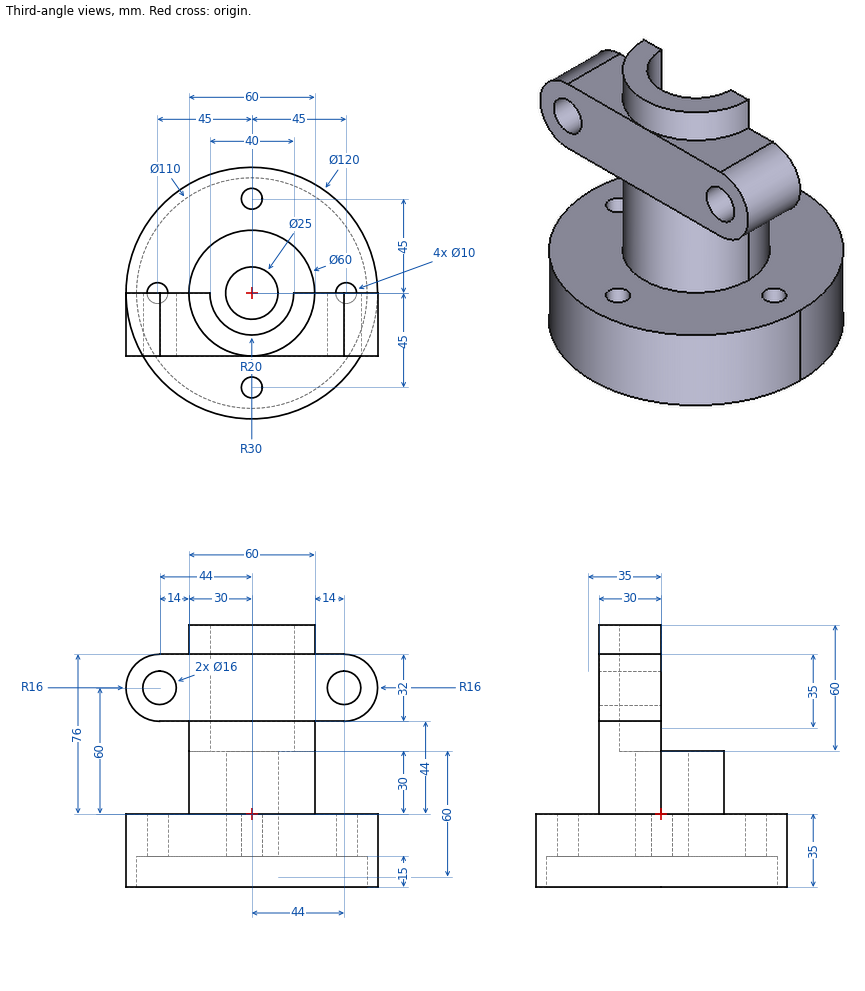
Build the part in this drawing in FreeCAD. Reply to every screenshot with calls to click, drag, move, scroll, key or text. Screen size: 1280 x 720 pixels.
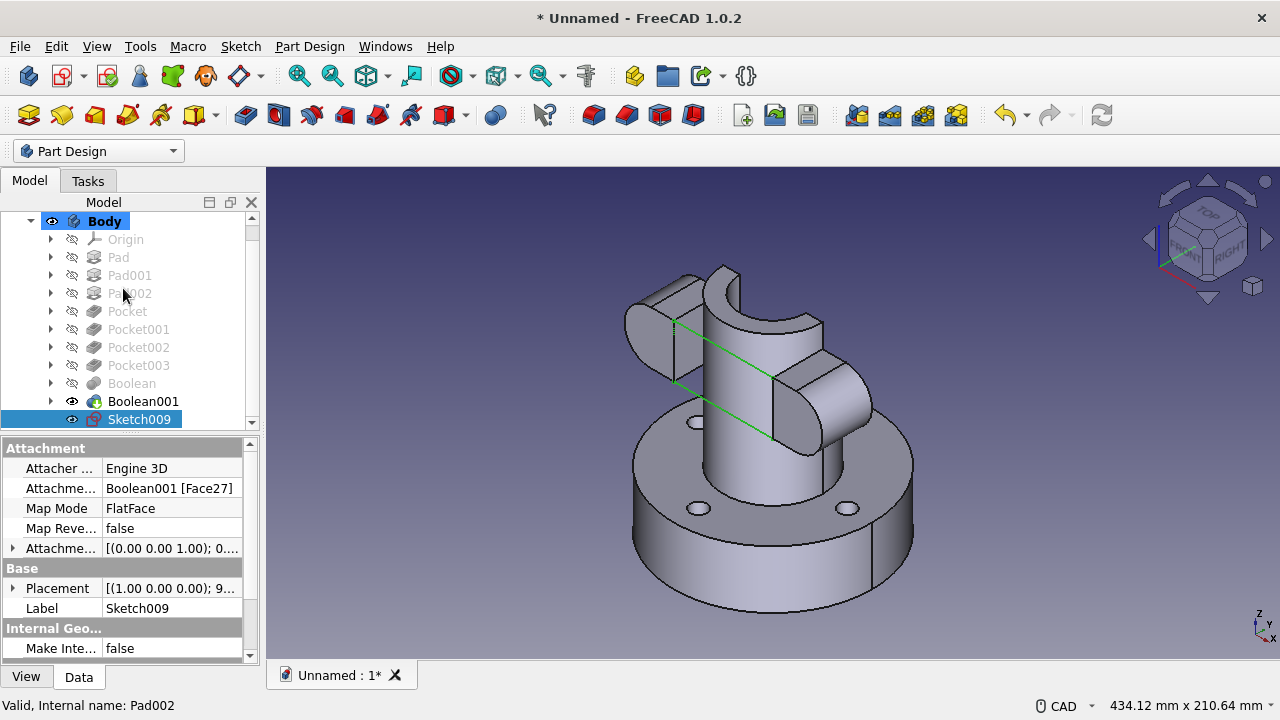
click(29, 116)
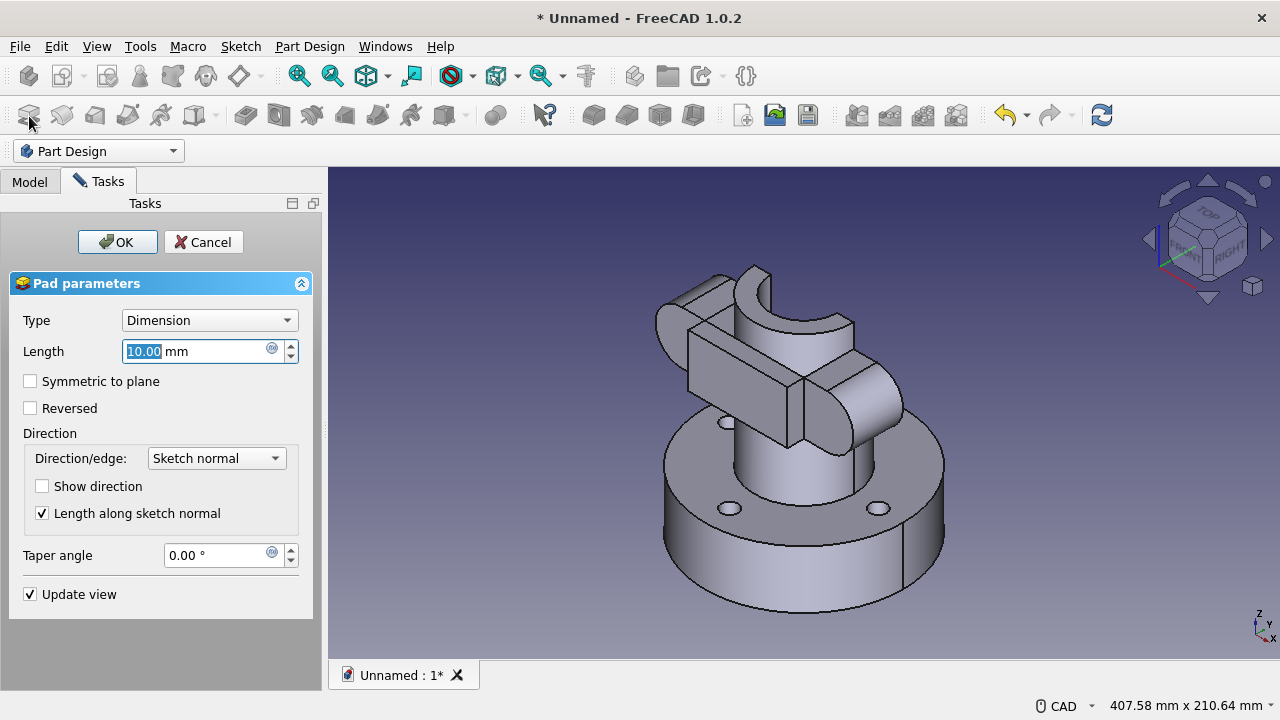
text(30)
key(Tab)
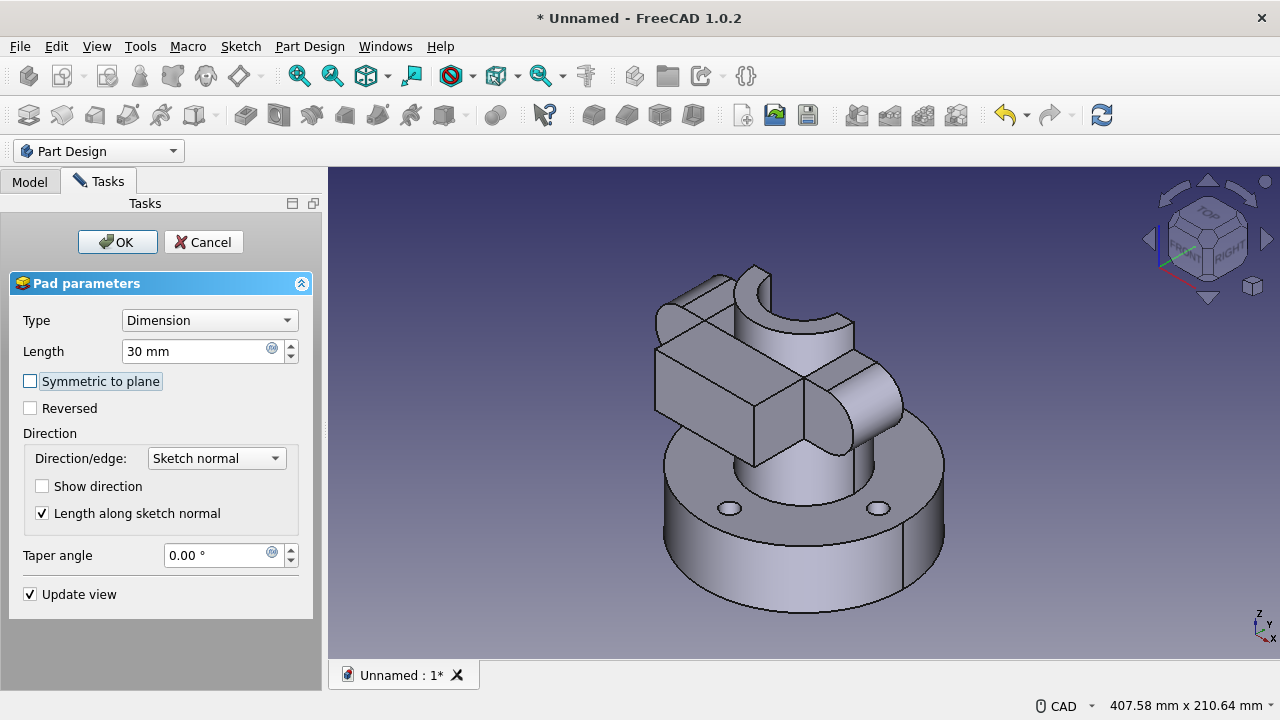
click(31, 408)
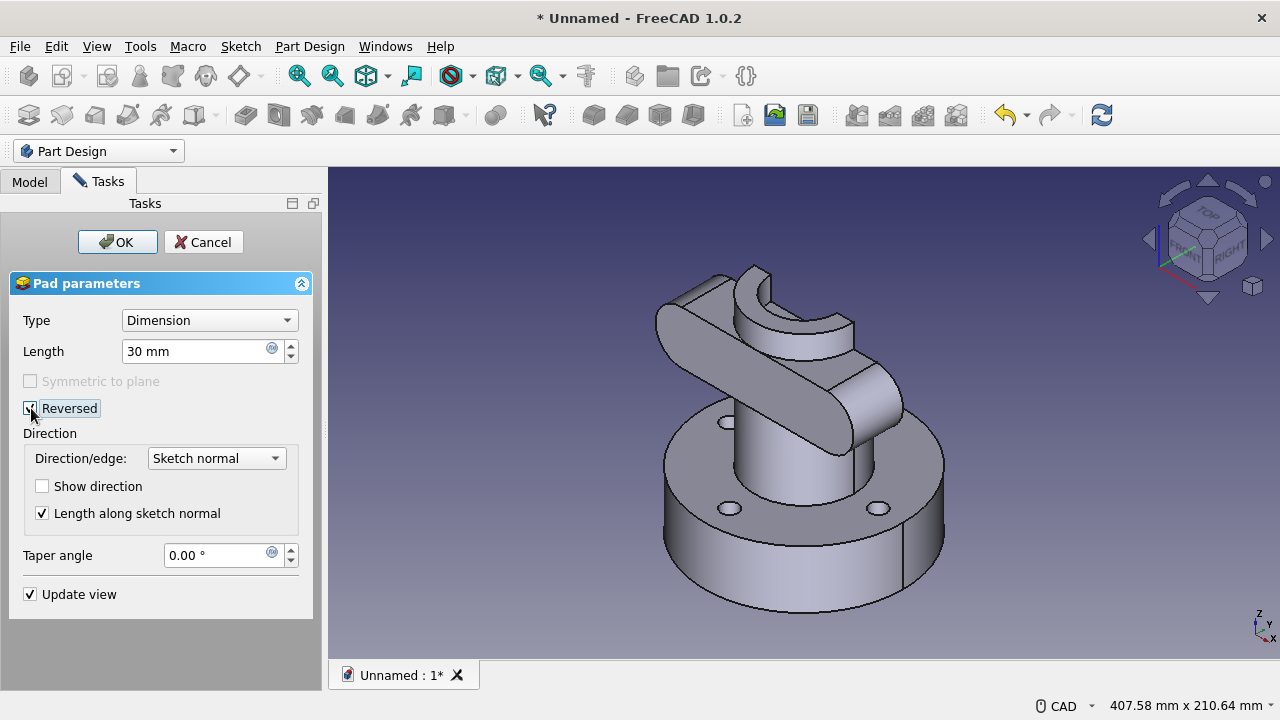
click(118, 242)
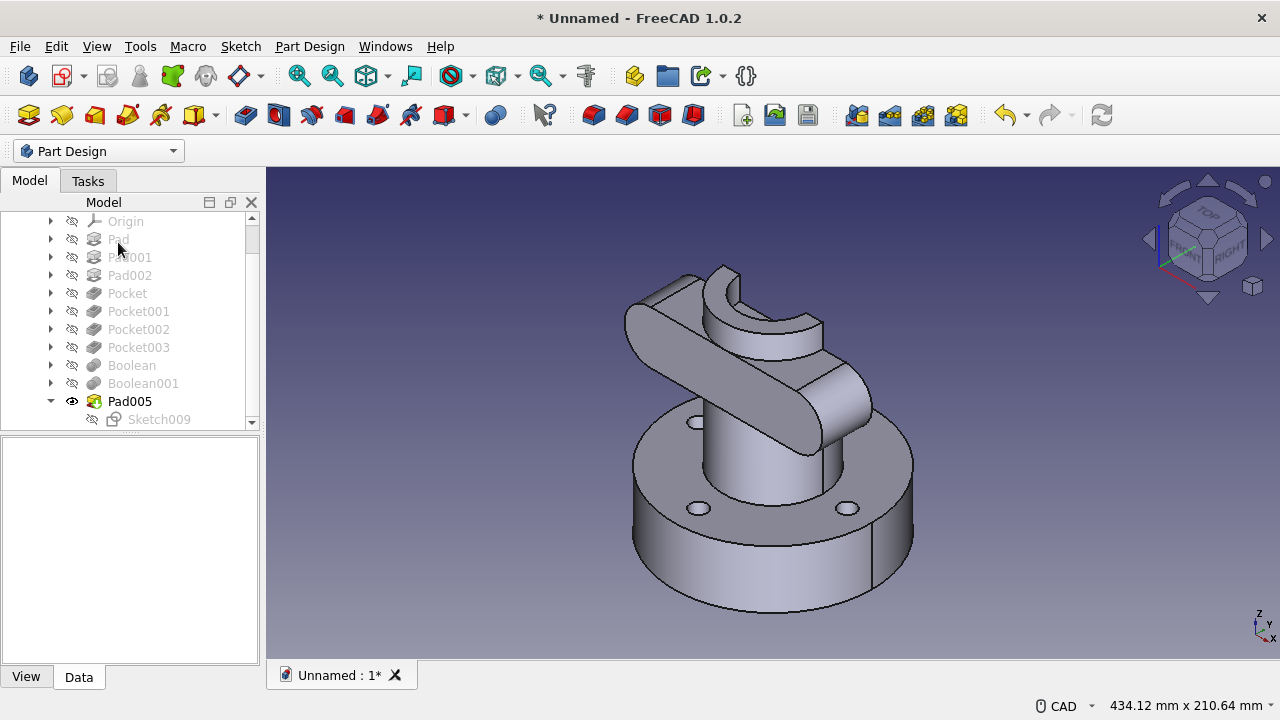
key(2)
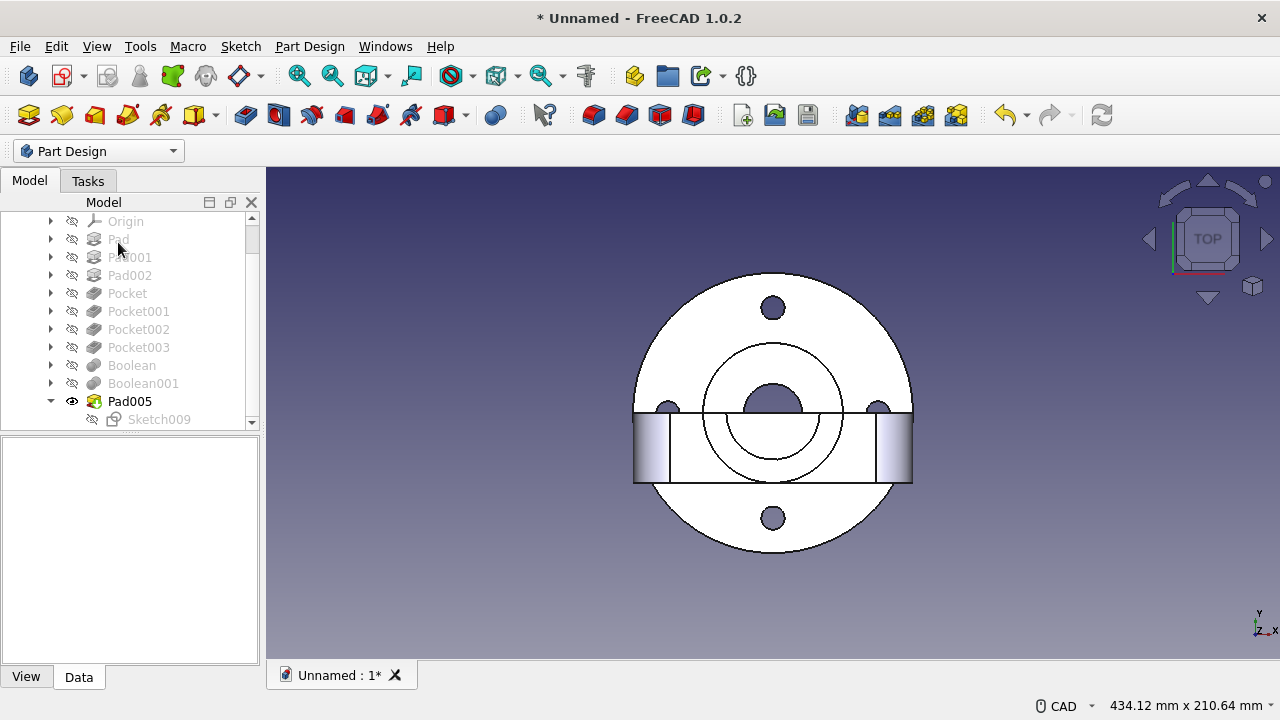
click(773, 435)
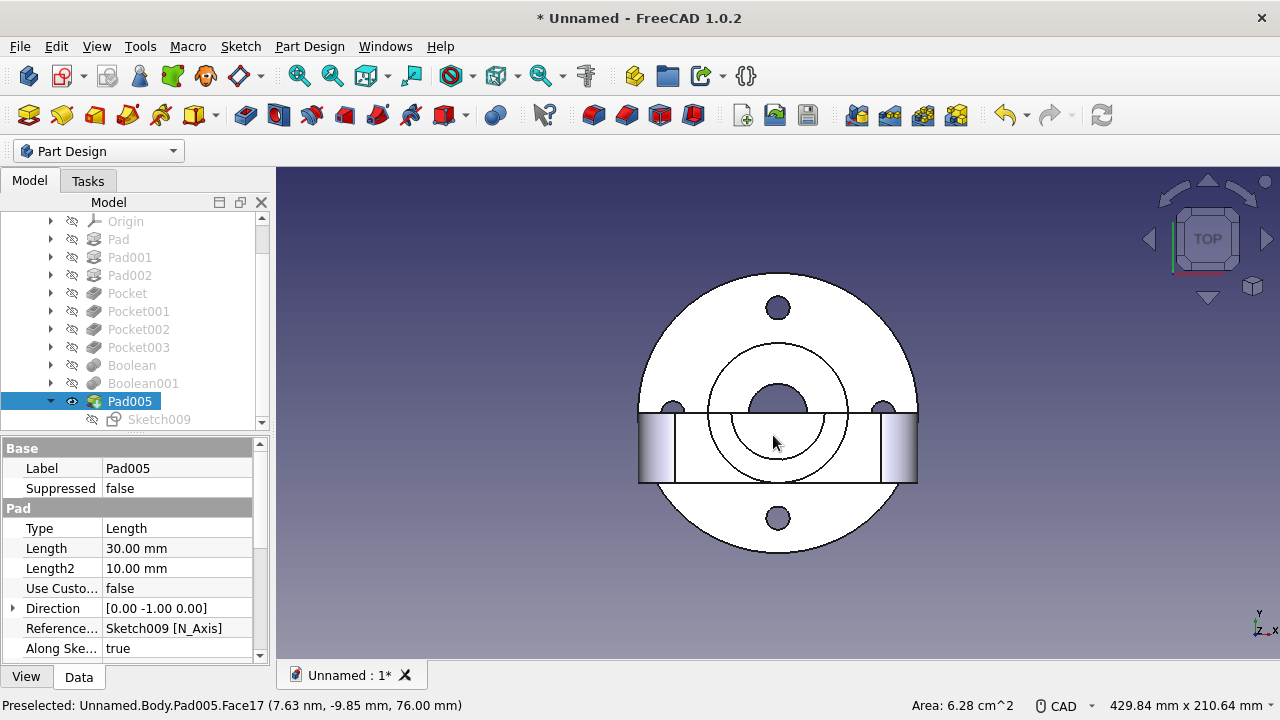
click(62, 76)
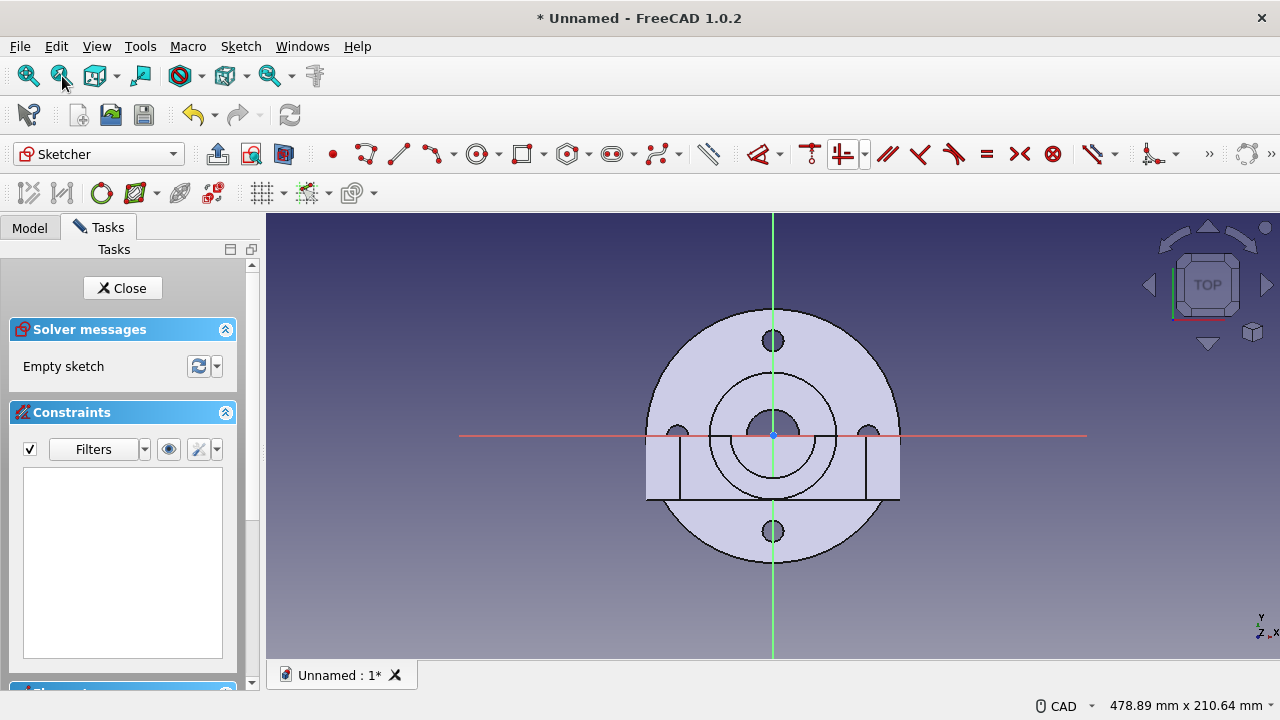
scroll(787, 461, up, 9)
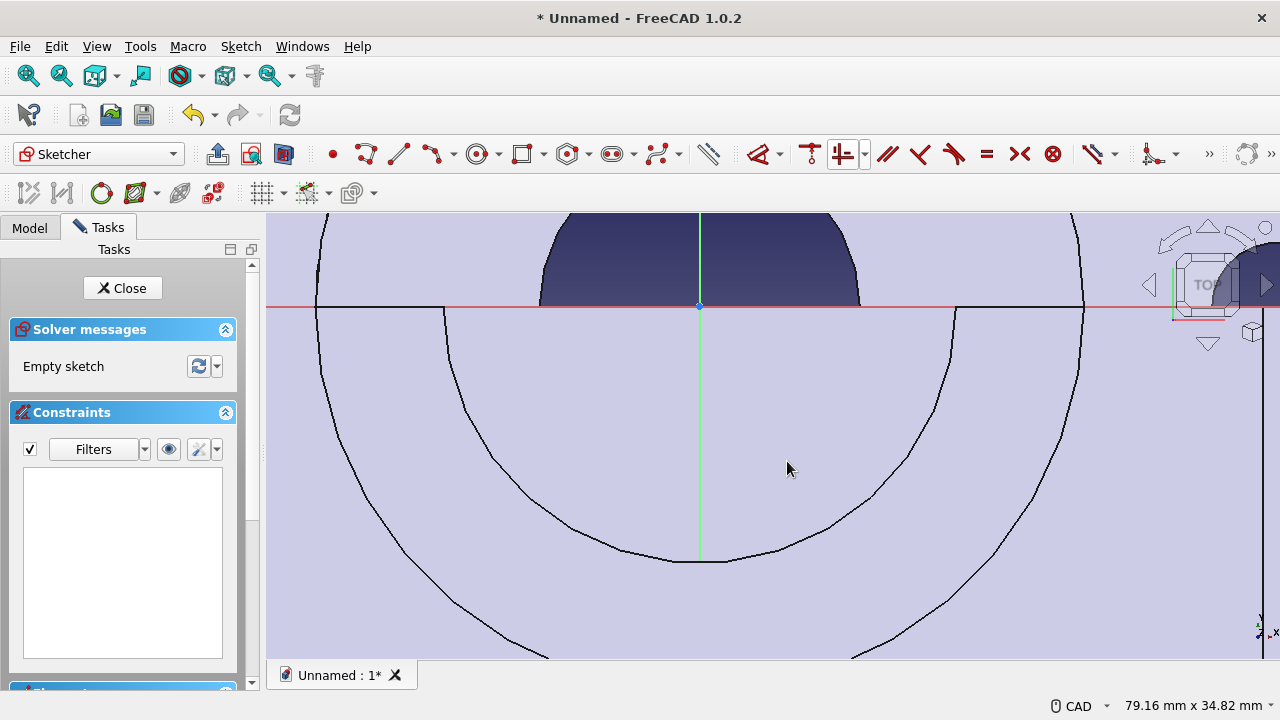
click(399, 154)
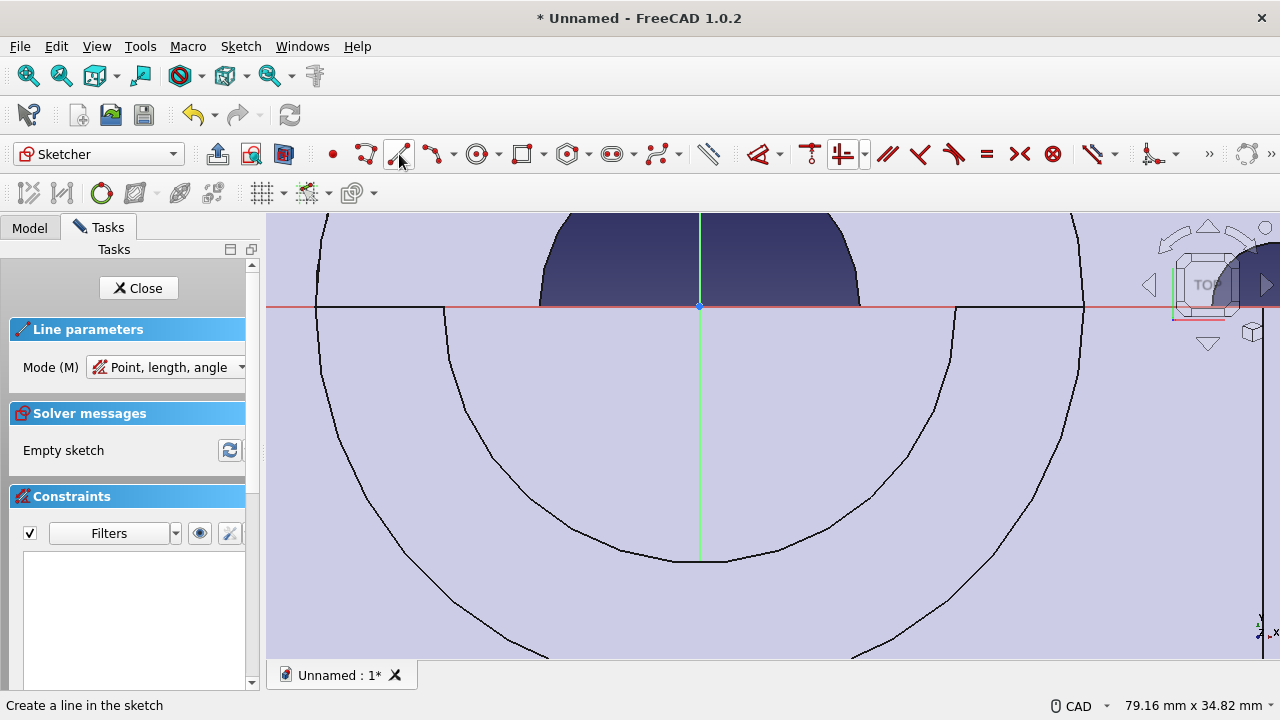
click(956, 307)
click(444, 316)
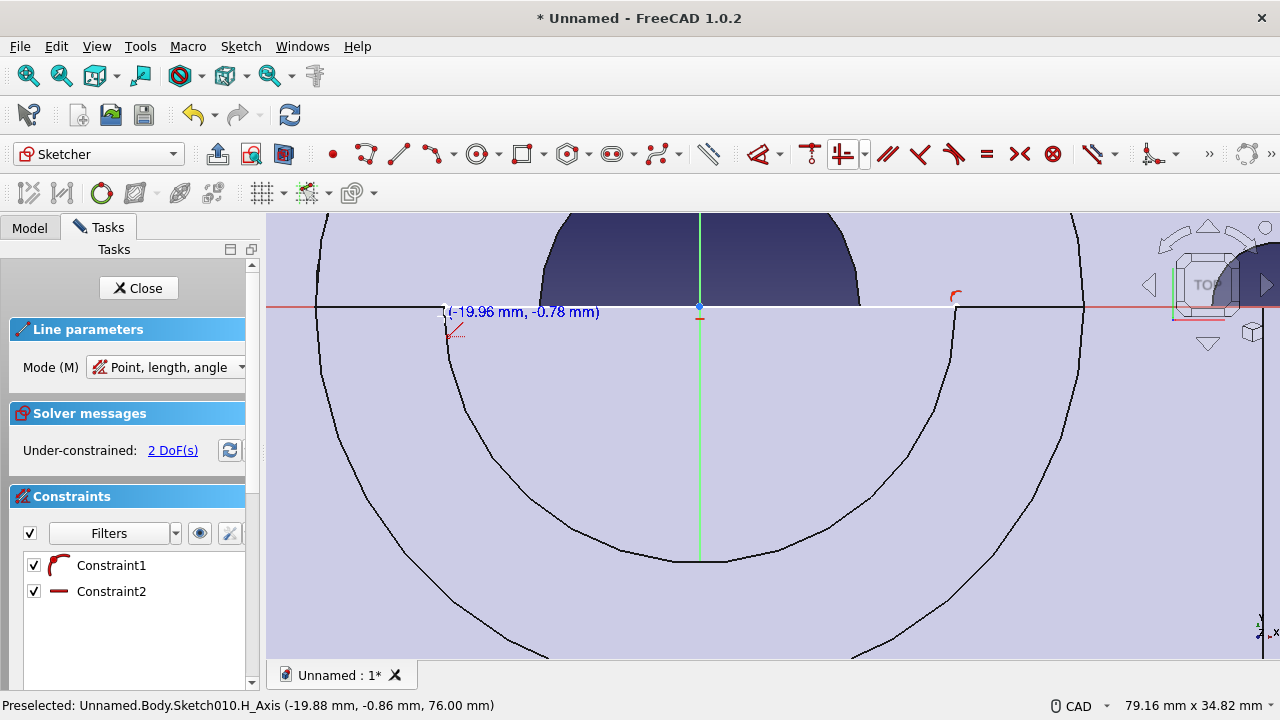
click(432, 154)